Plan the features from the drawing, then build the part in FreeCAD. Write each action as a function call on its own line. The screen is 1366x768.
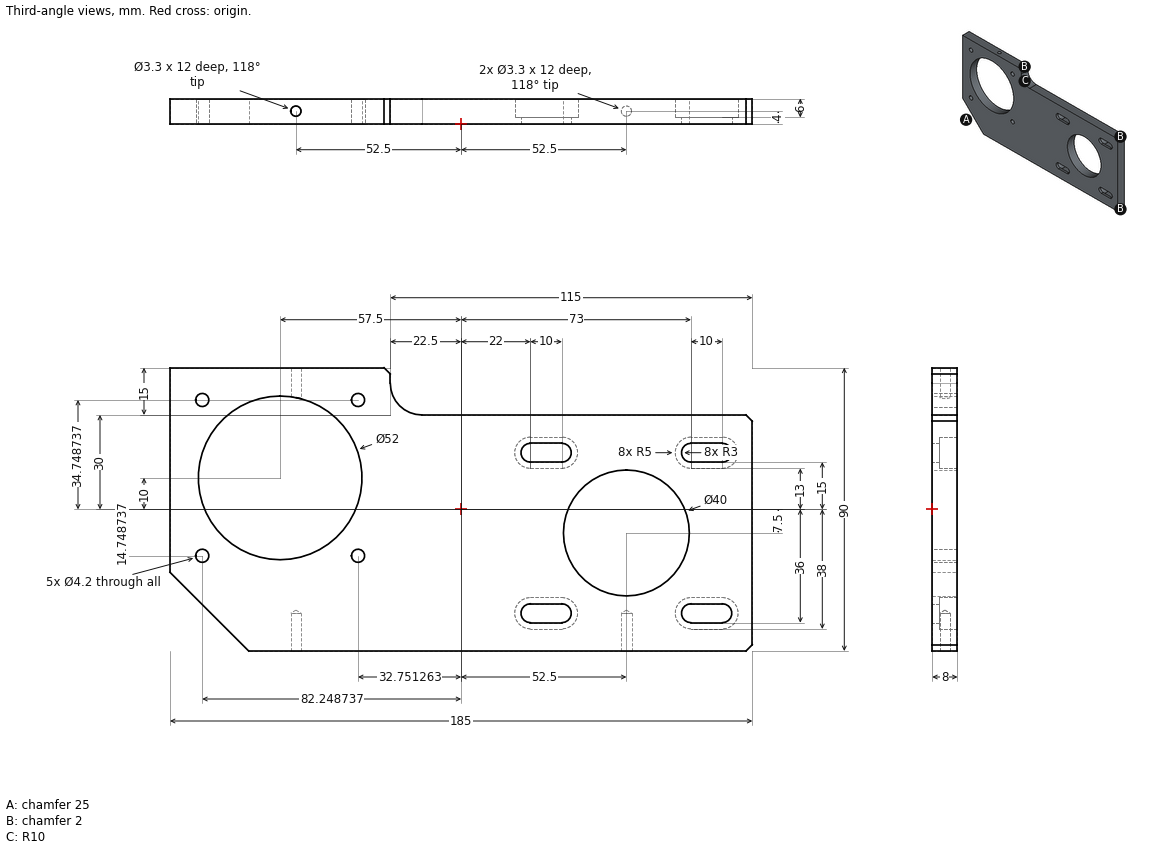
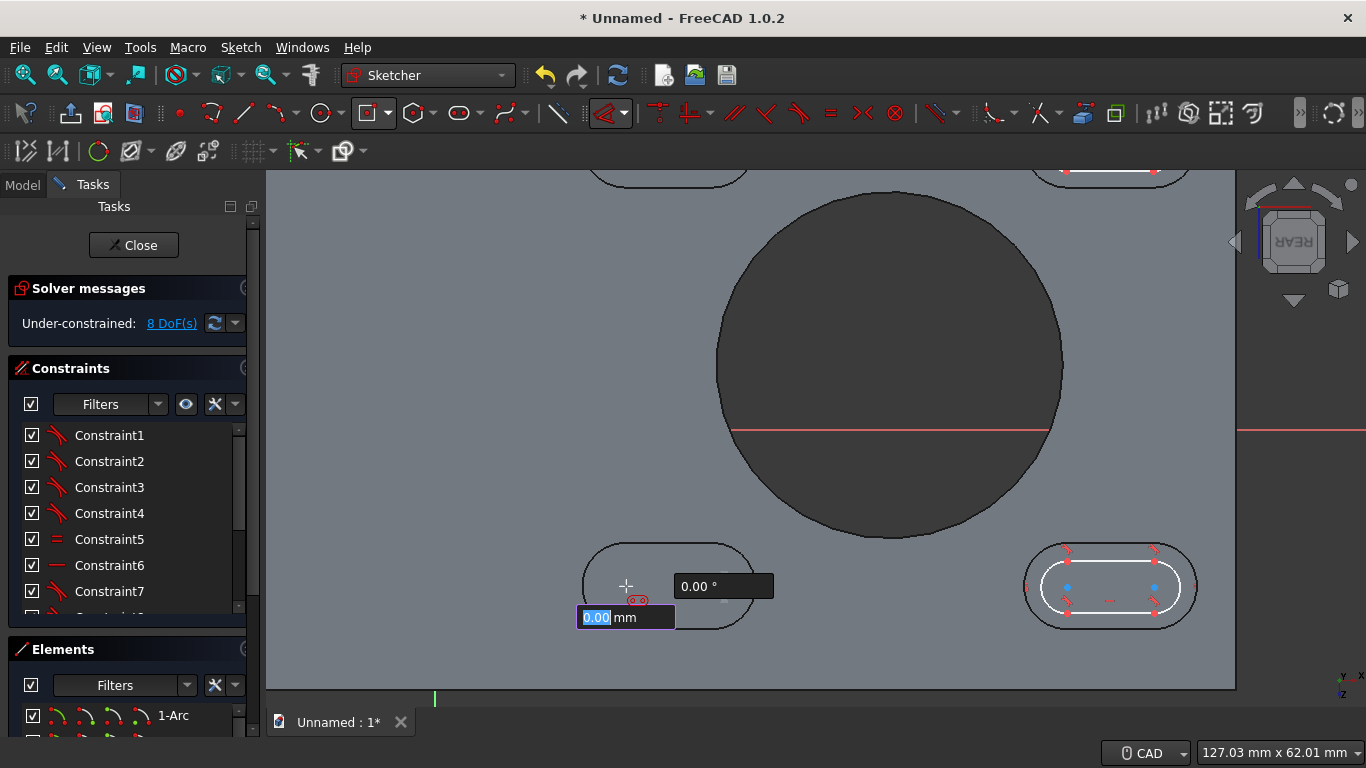
click(712, 586)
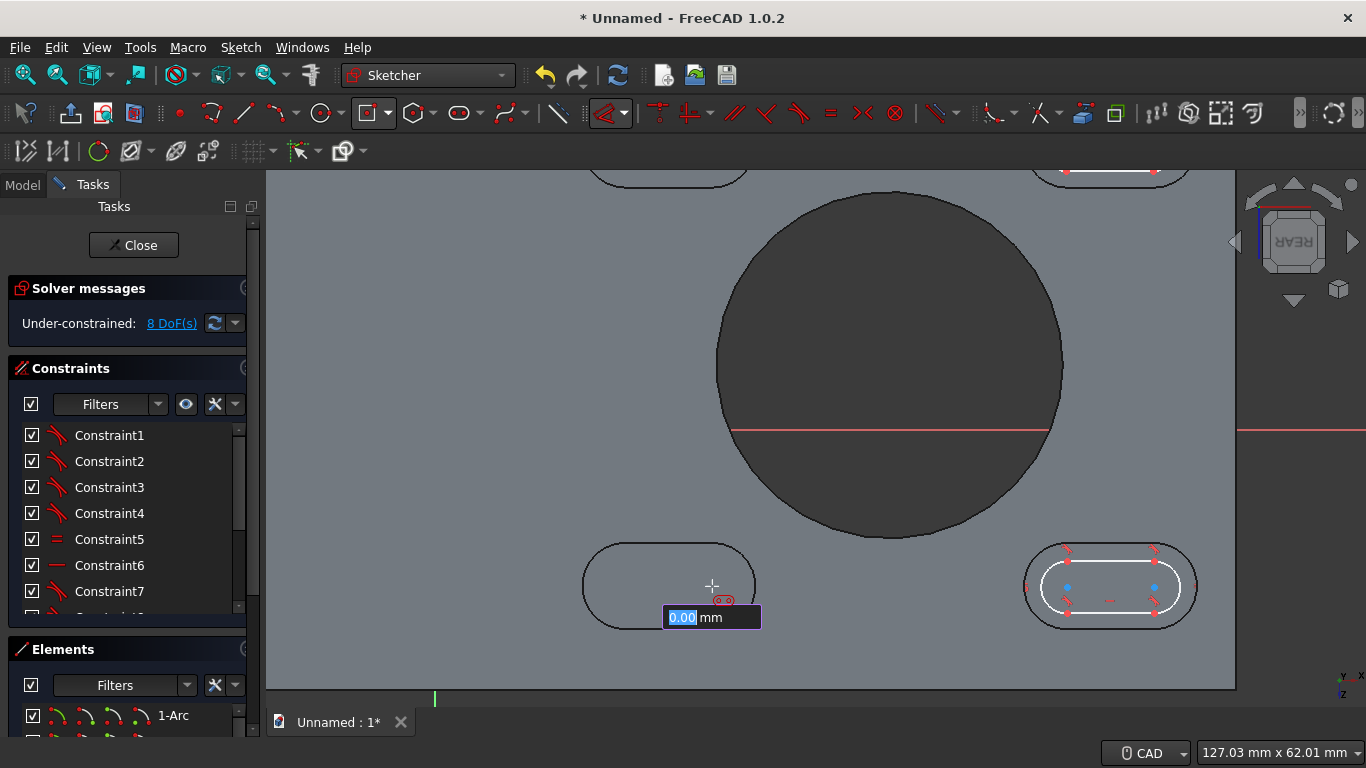
click(669, 560)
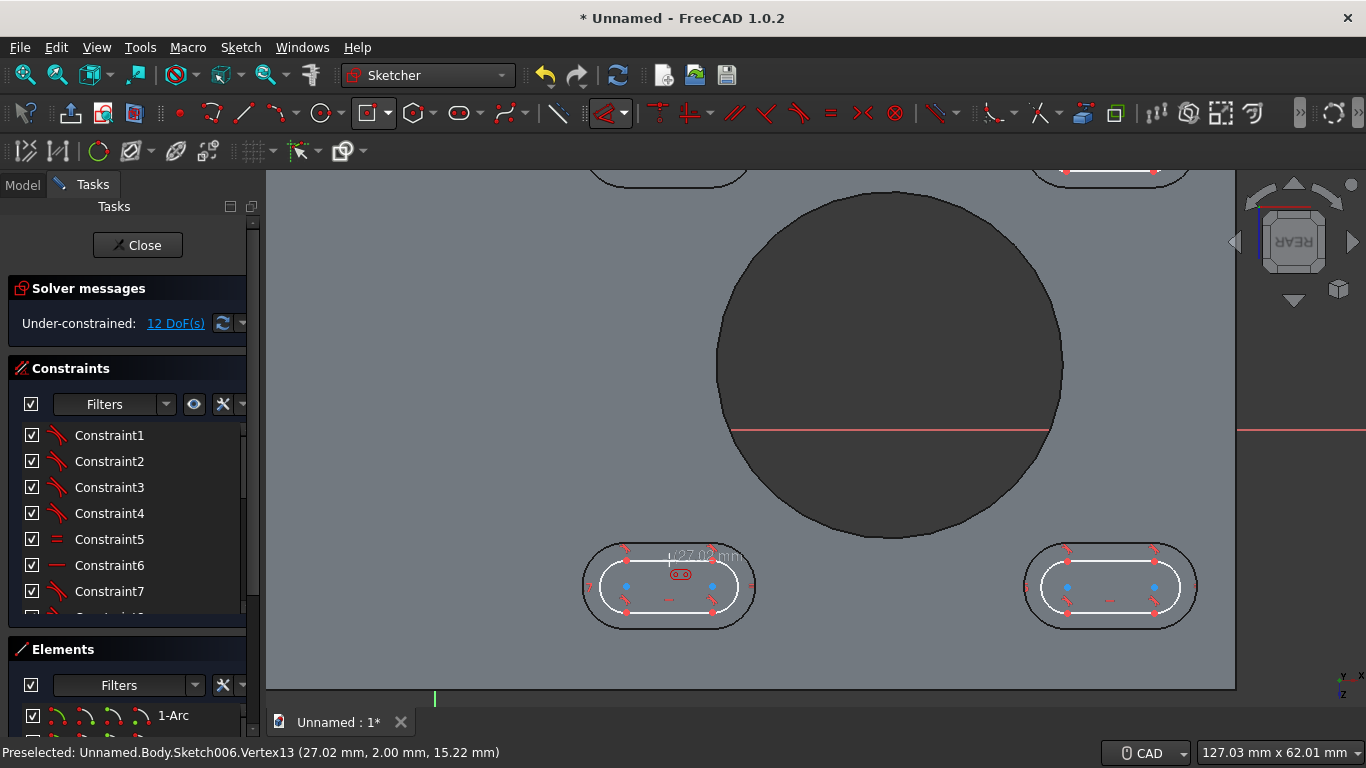
scroll(626, 587, down, 2)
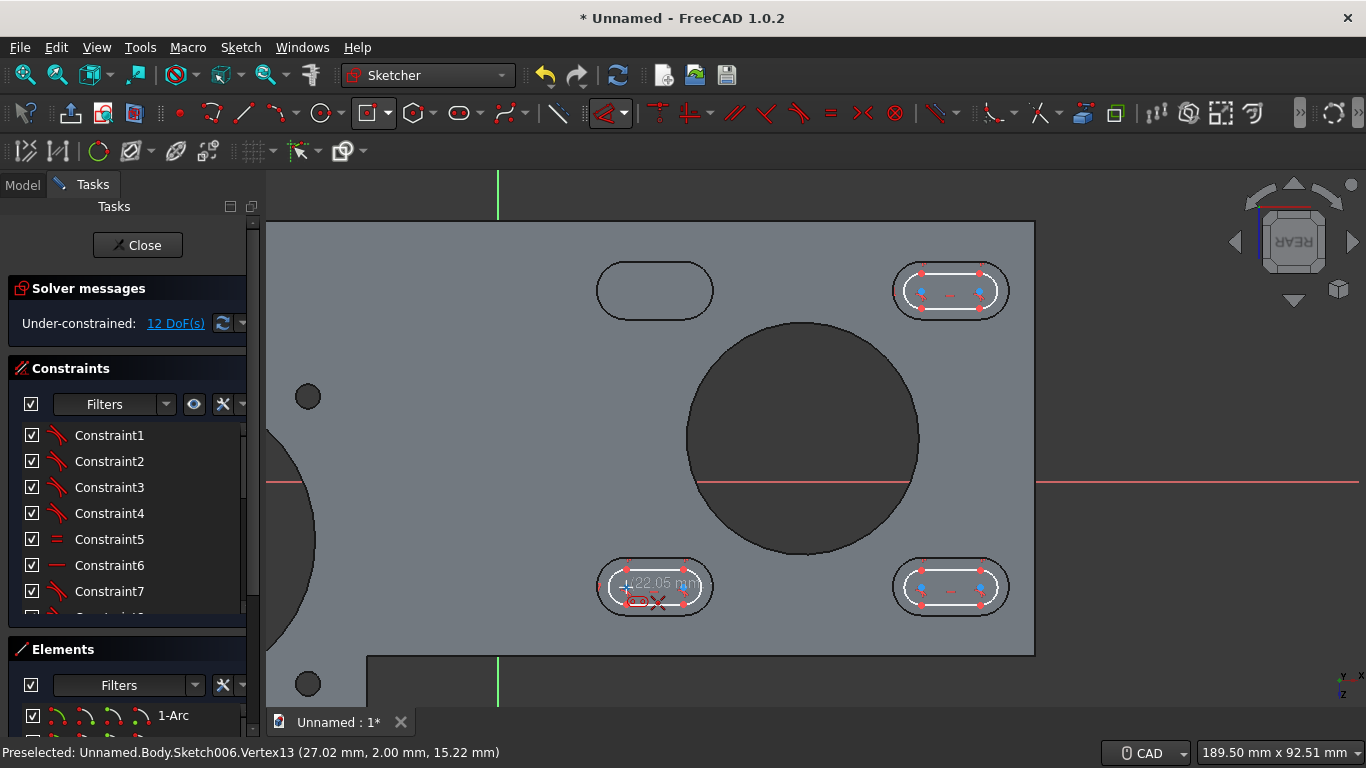
scroll(626, 291, up, 2)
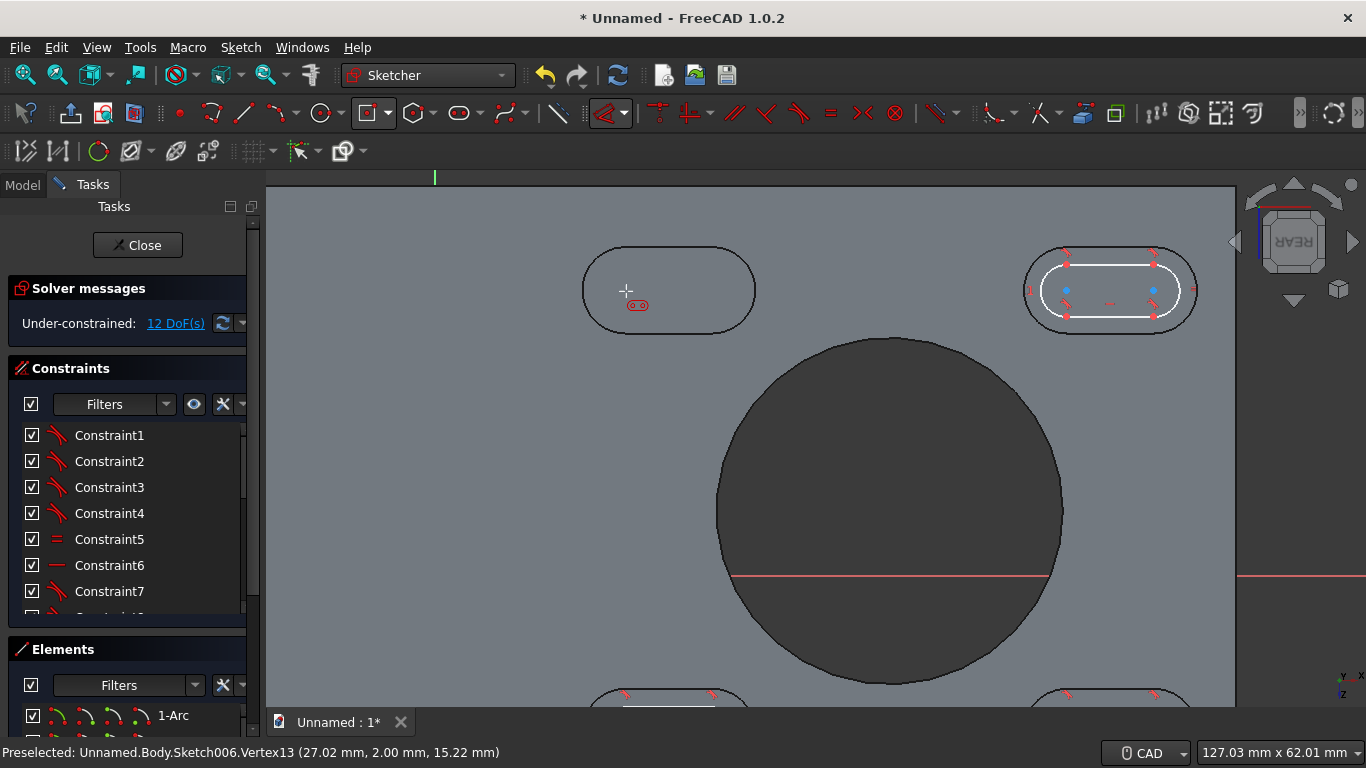
click(626, 290)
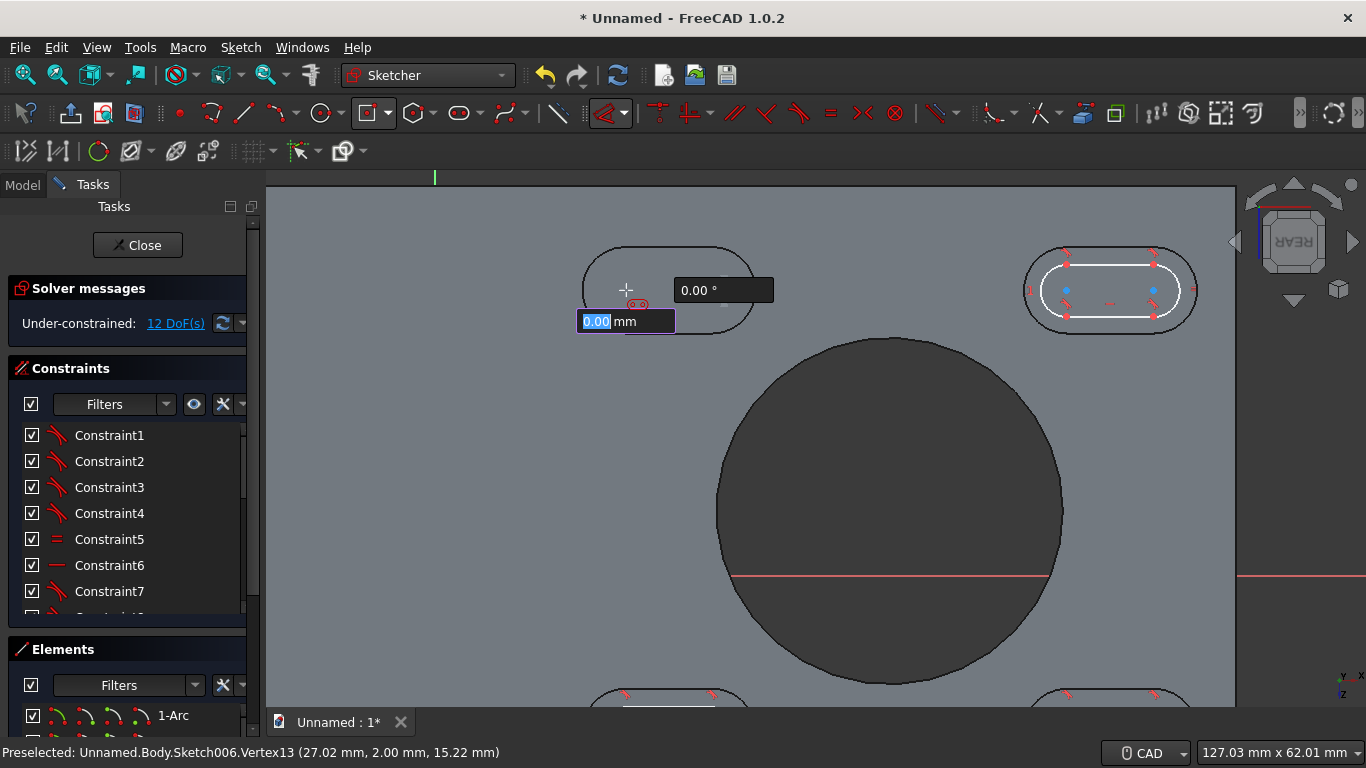
click(712, 290)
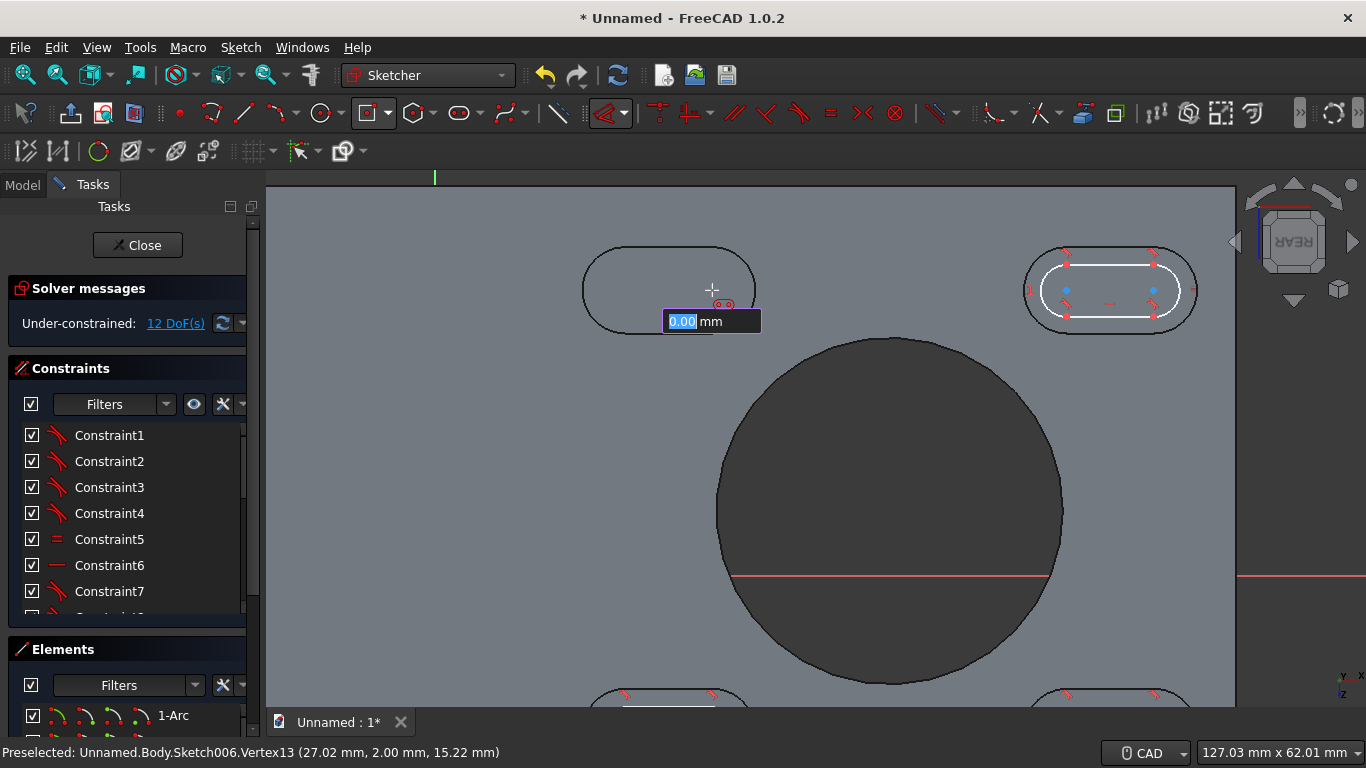
click(669, 316)
key(Escape)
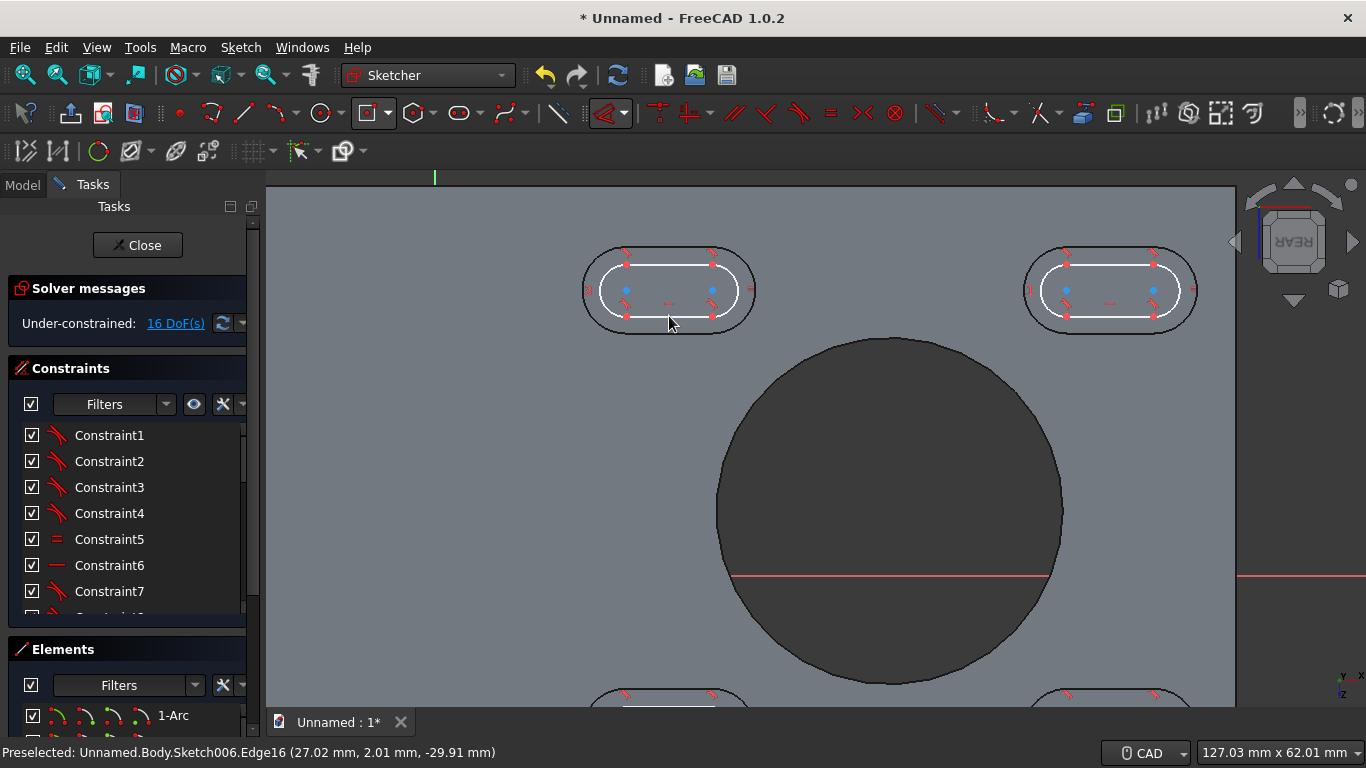
scroll(626, 291, down, 2)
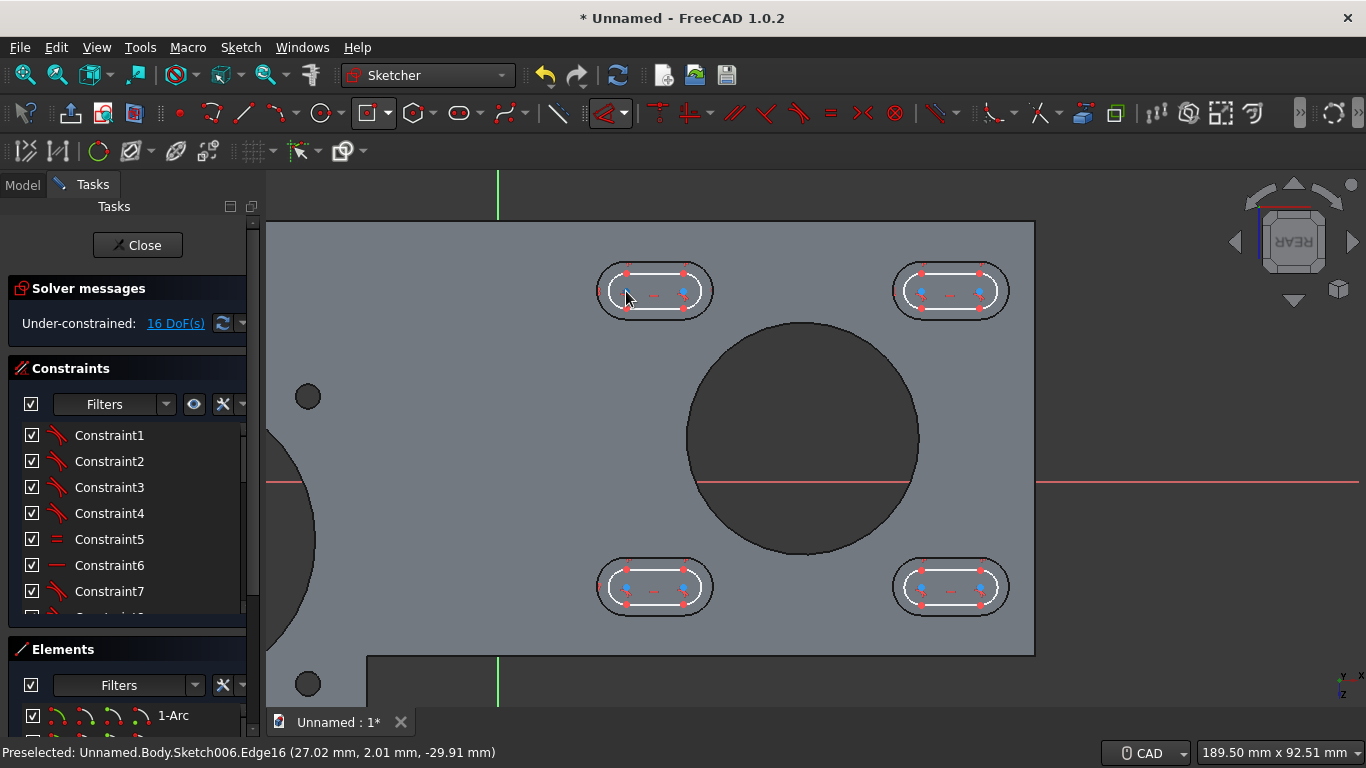
click(908, 577)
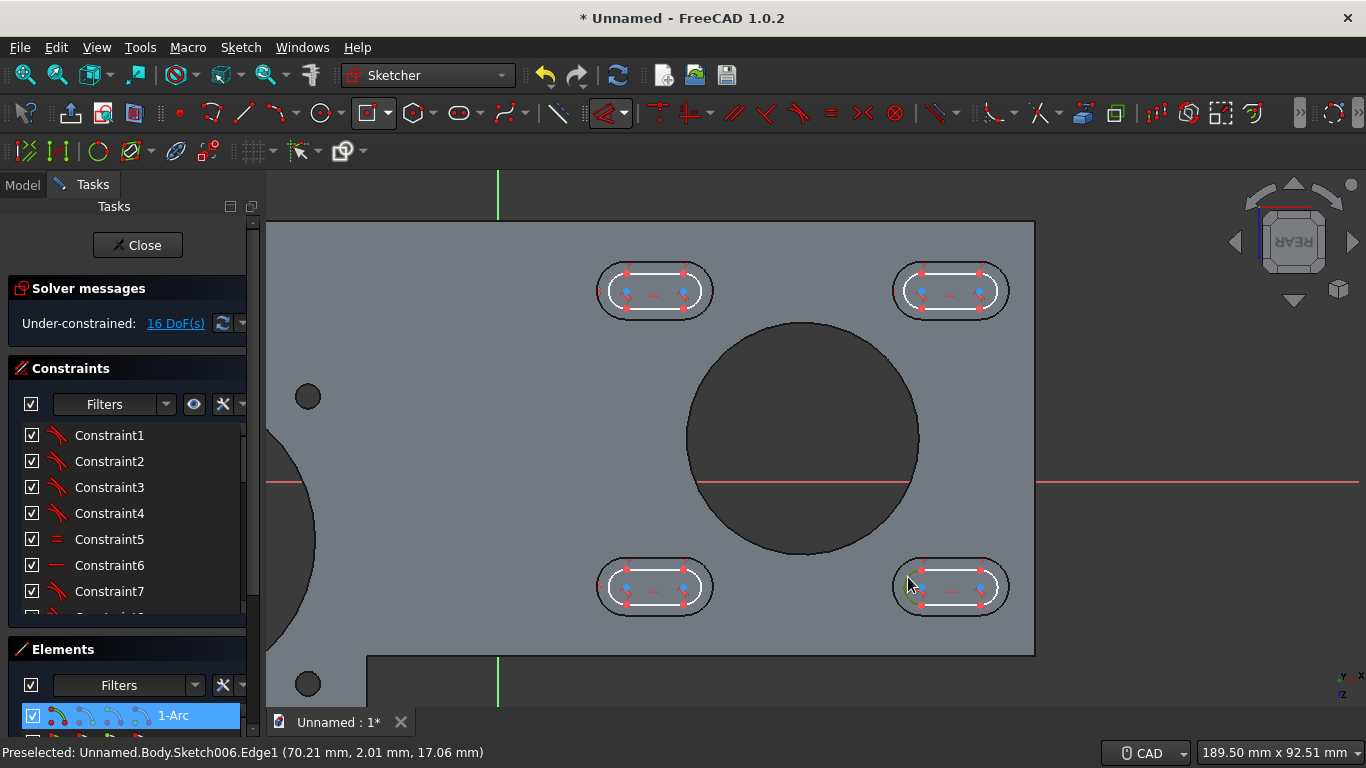
click(907, 281)